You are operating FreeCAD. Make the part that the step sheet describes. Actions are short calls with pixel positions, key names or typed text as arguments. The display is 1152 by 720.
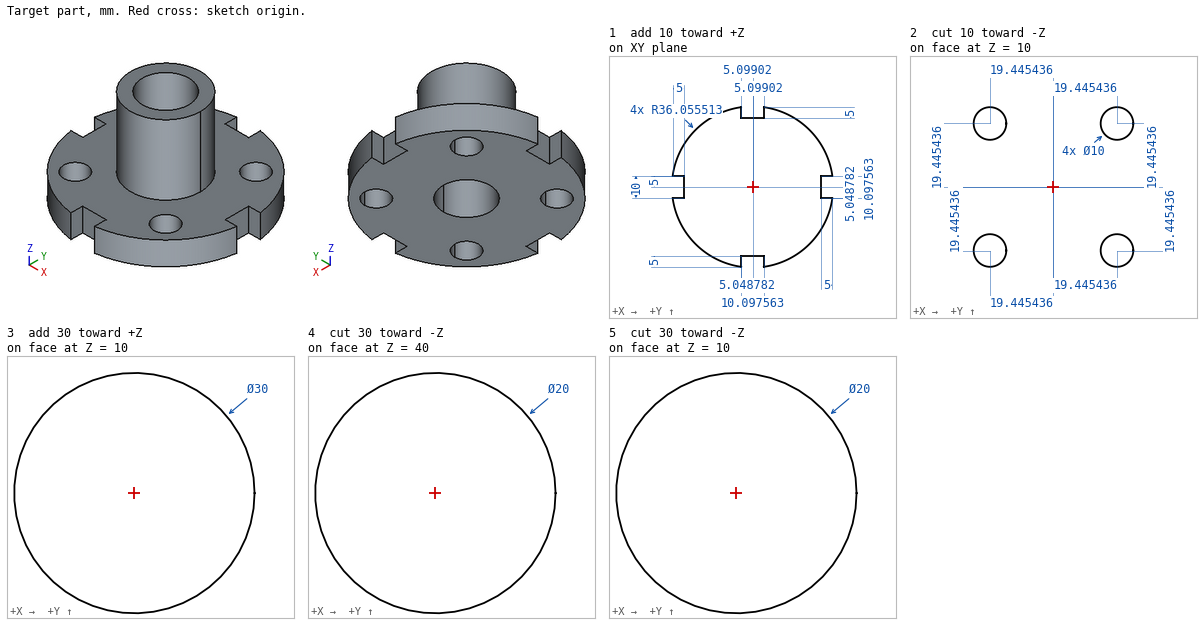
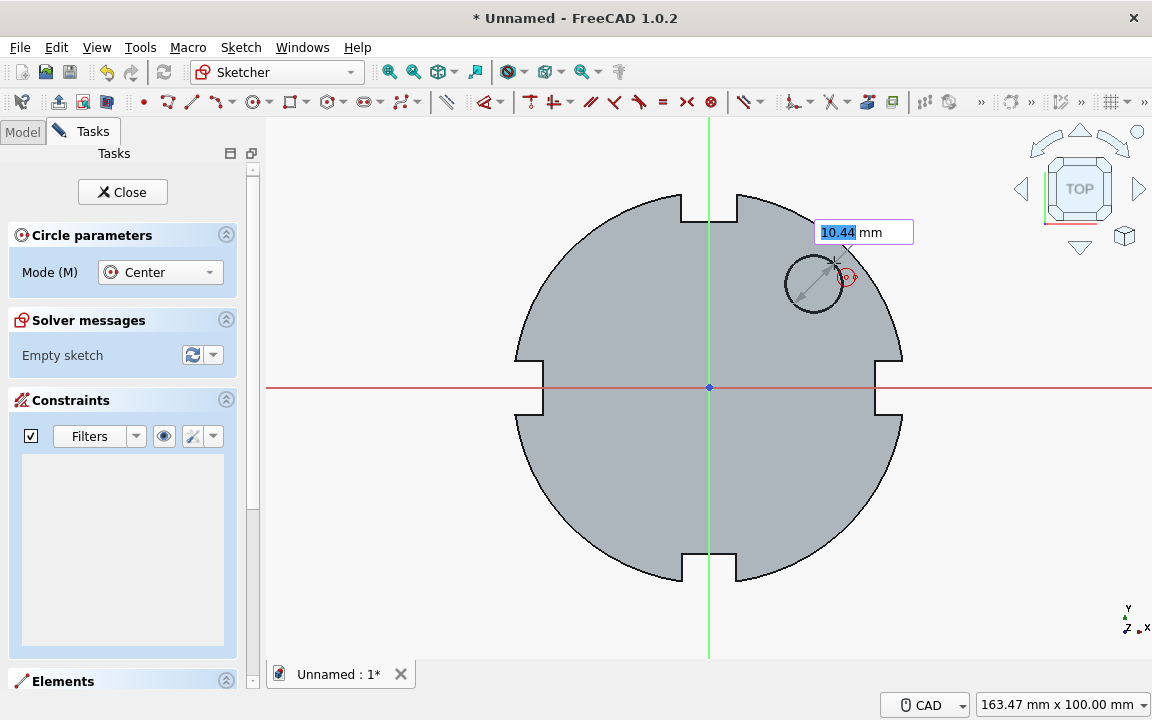
text(10)
key(Return)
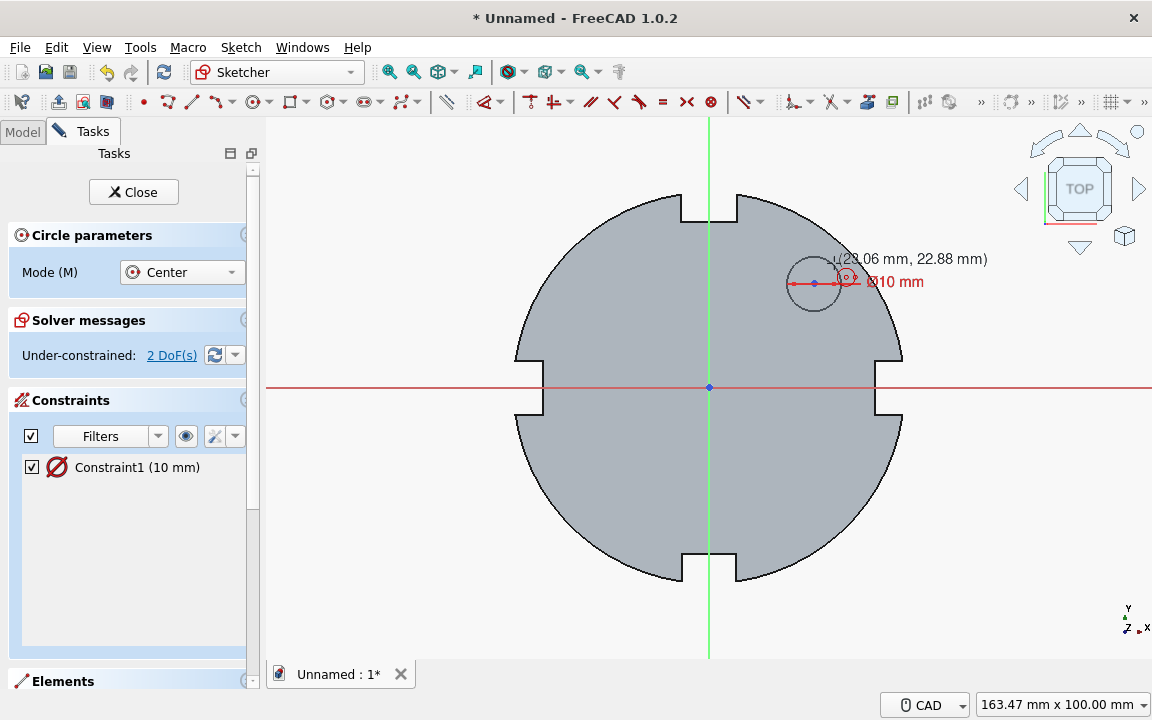
click(814, 493)
move(834, 474)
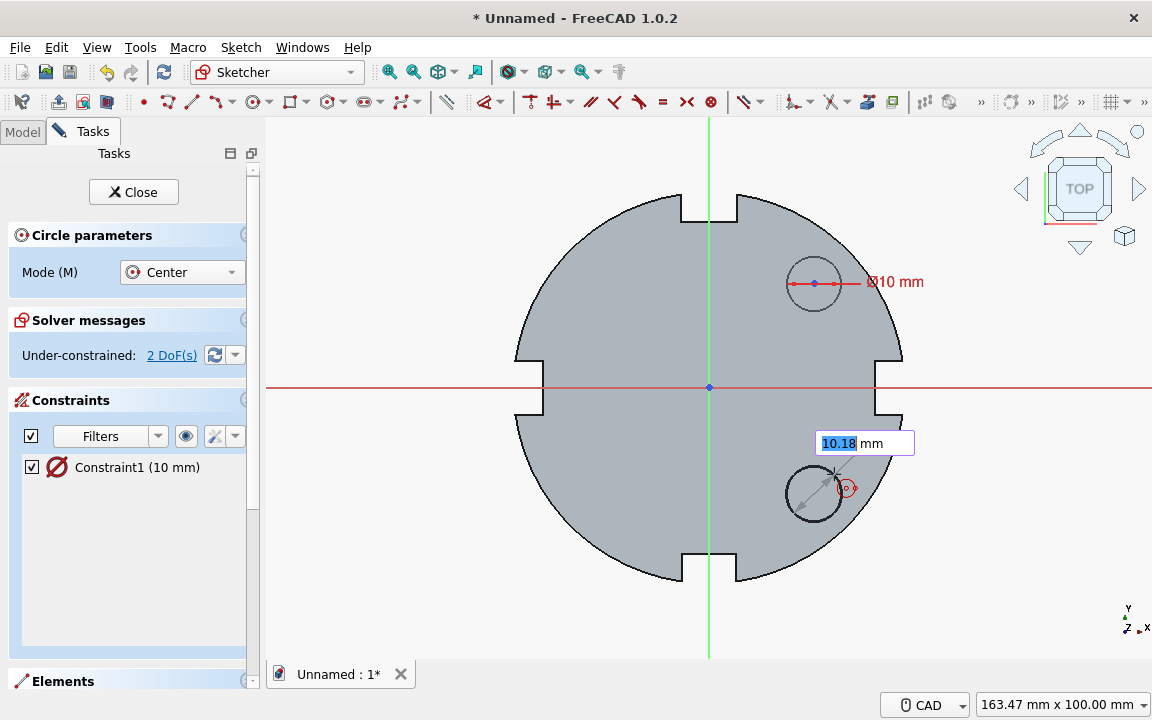
text(10)
key(Return)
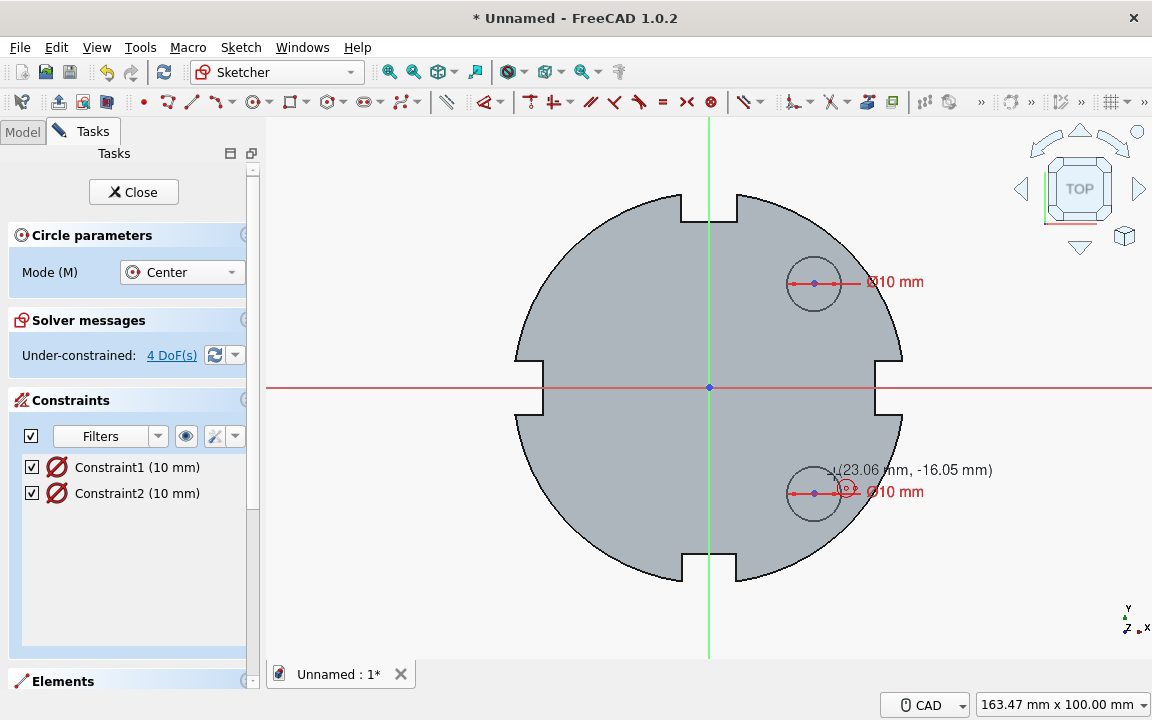
click(604, 493)
move(623, 474)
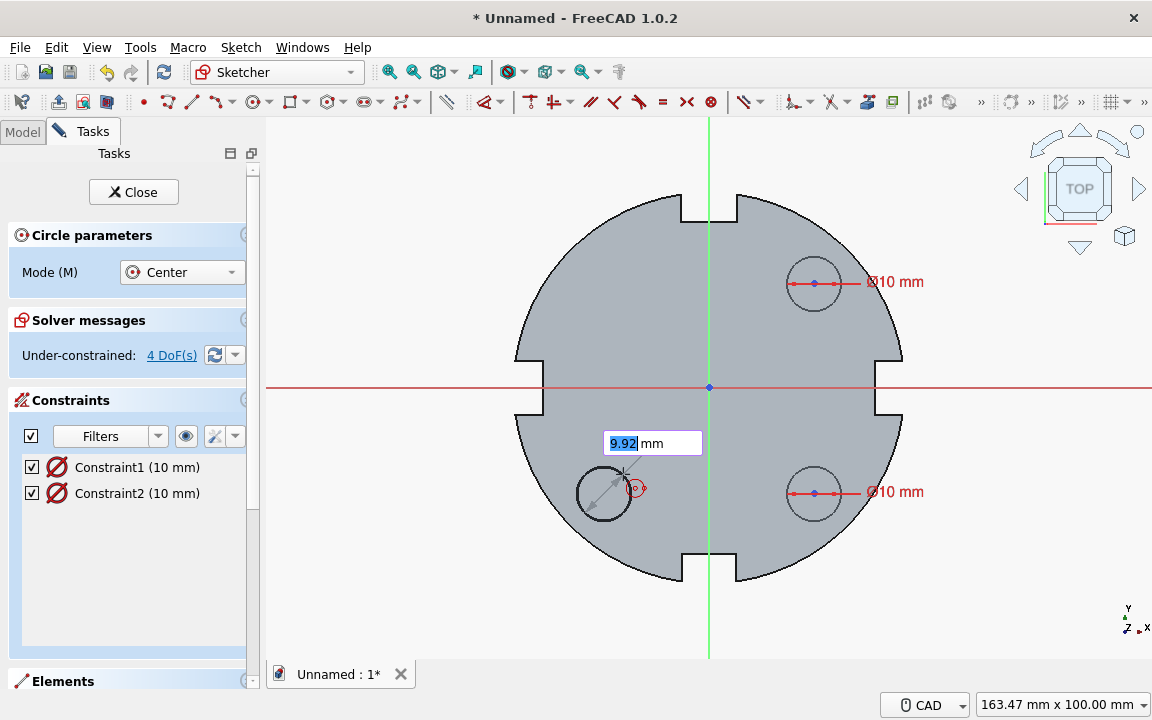
text(10)
key(Return)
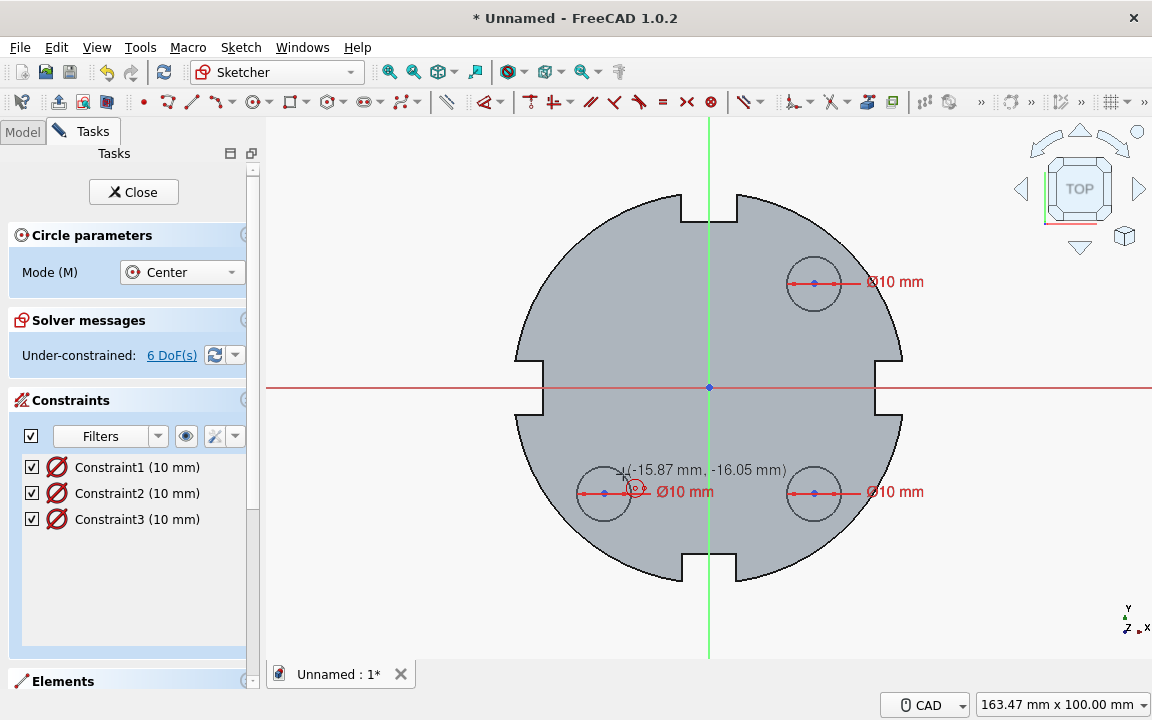
click(604, 283)
move(623, 263)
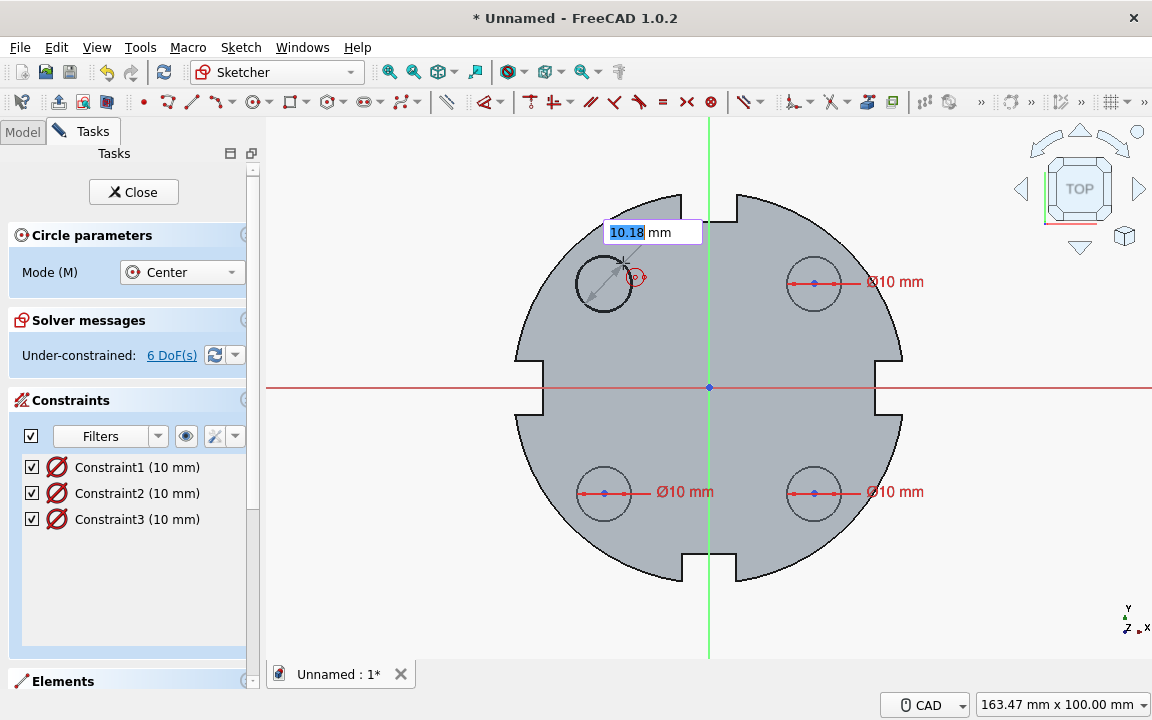
text(10)
key(Return)
key(Escape)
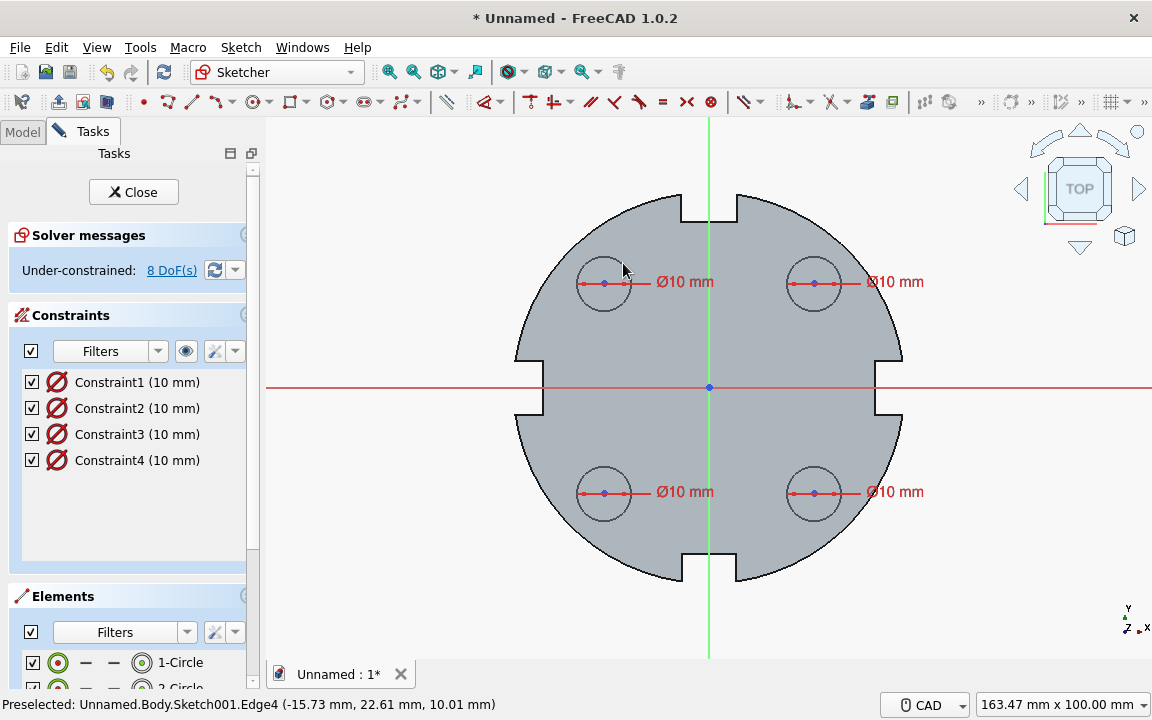
click(484, 102)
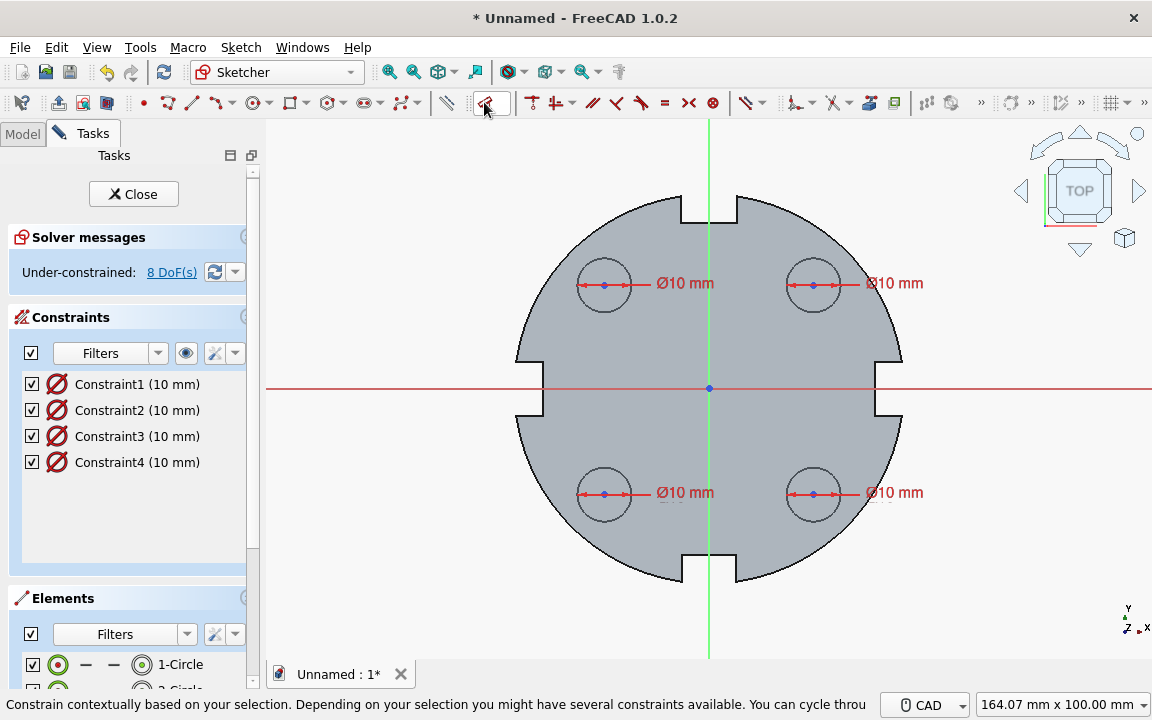
click(814, 285)
click(761, 251)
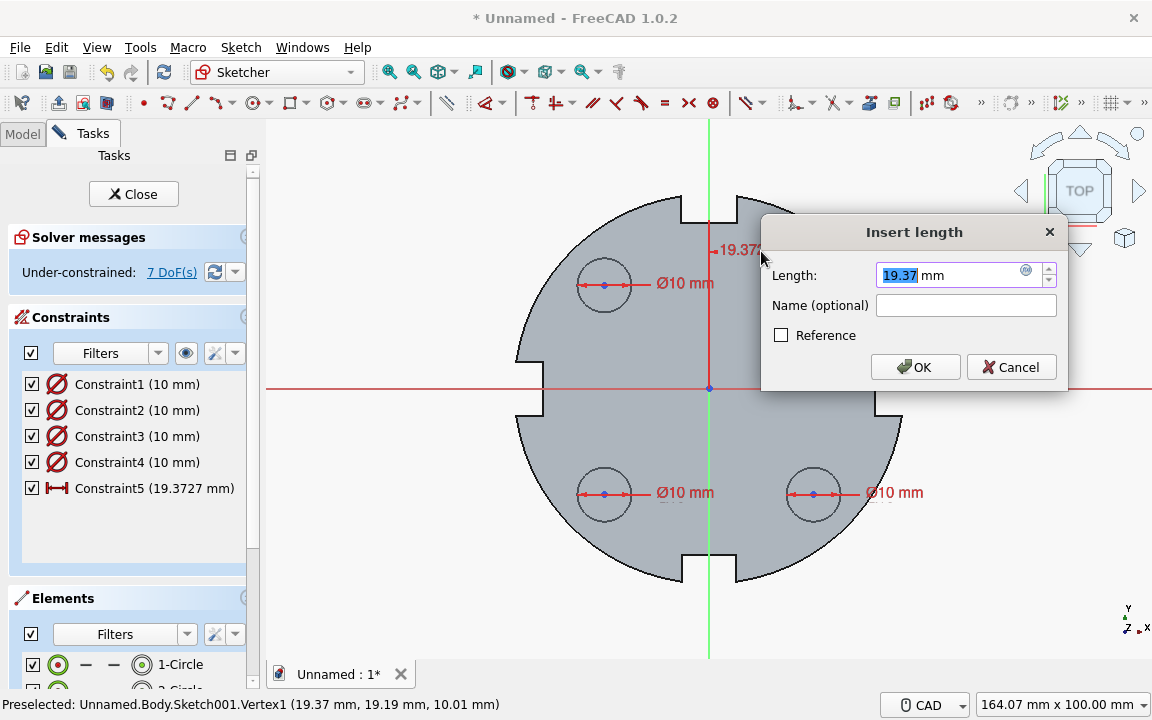
text(19.445436)
key(Return)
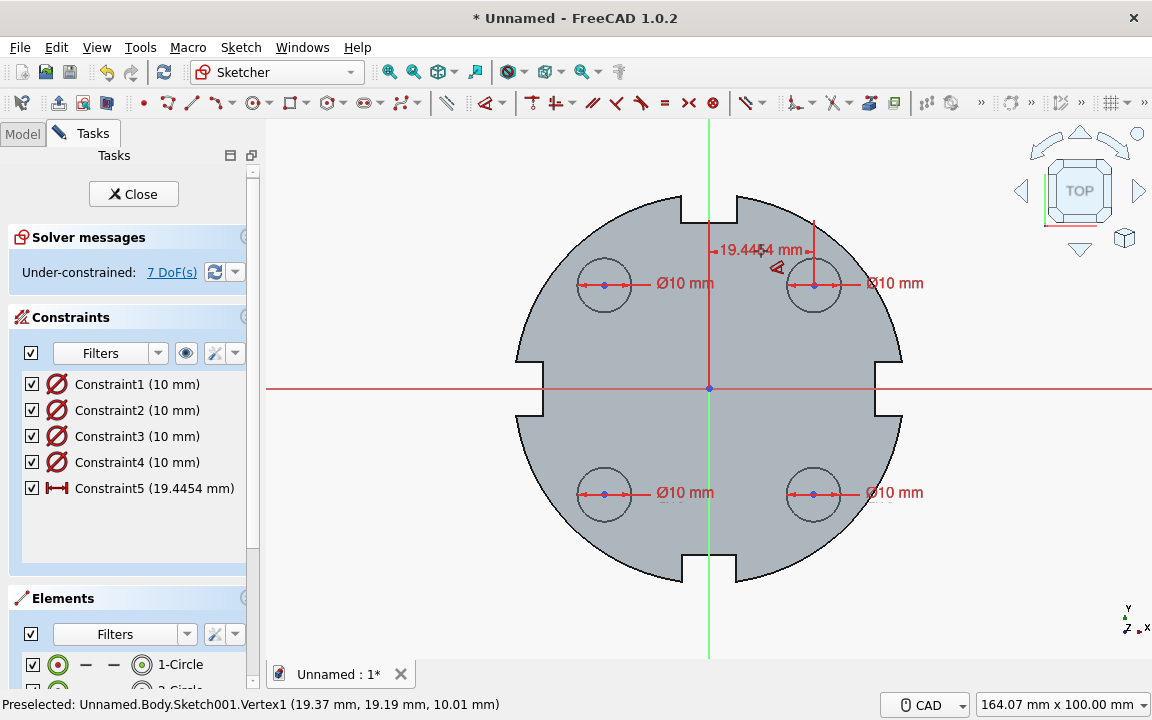
click(814, 285)
click(848, 337)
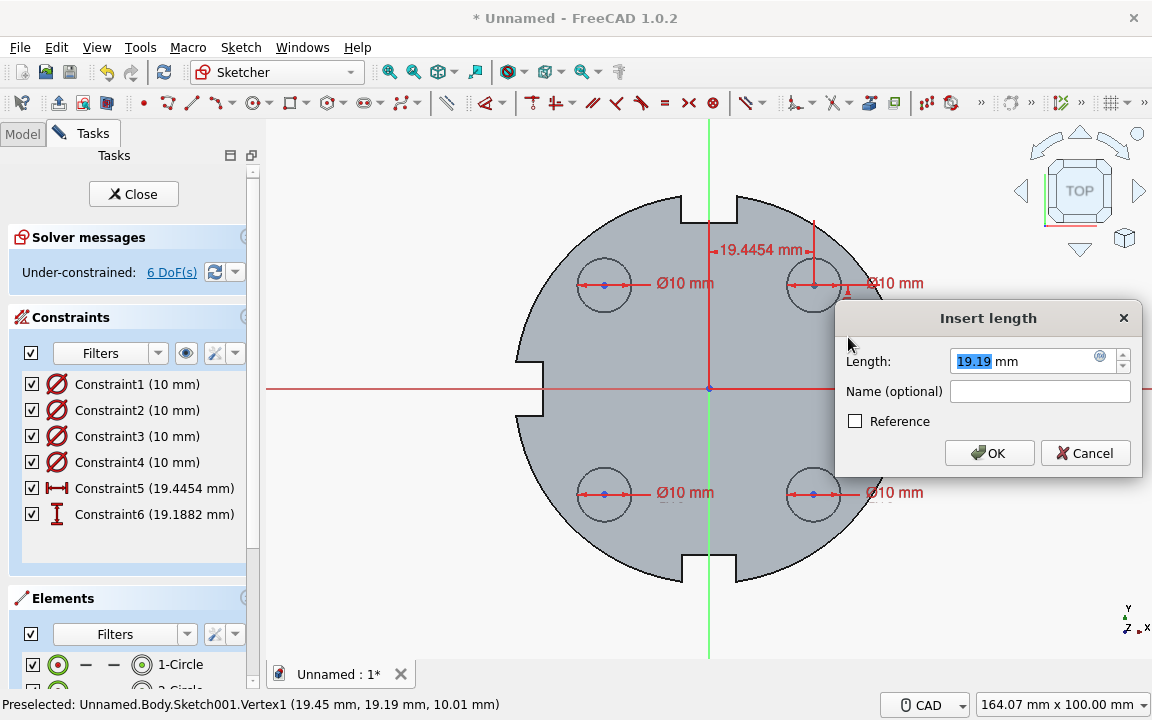
text(19.445436)
key(Return)